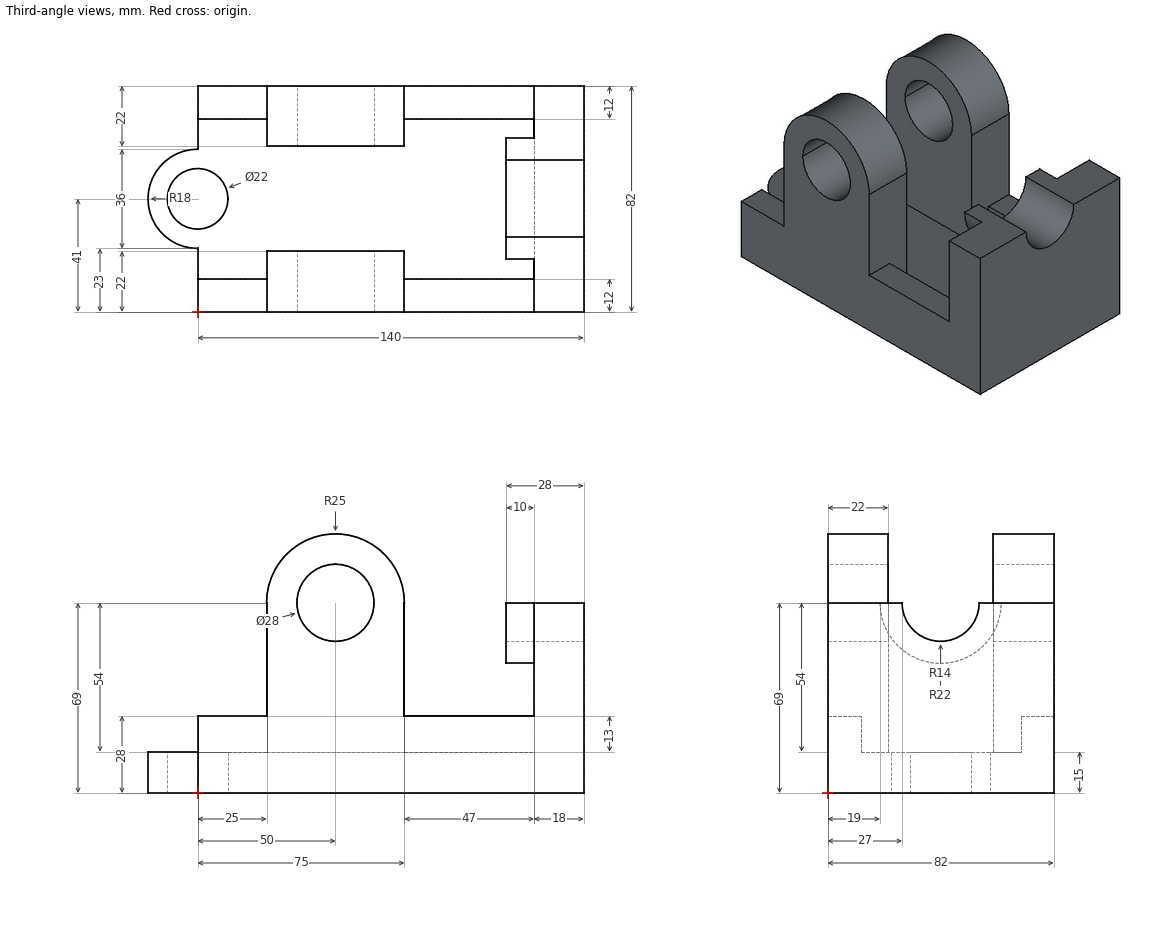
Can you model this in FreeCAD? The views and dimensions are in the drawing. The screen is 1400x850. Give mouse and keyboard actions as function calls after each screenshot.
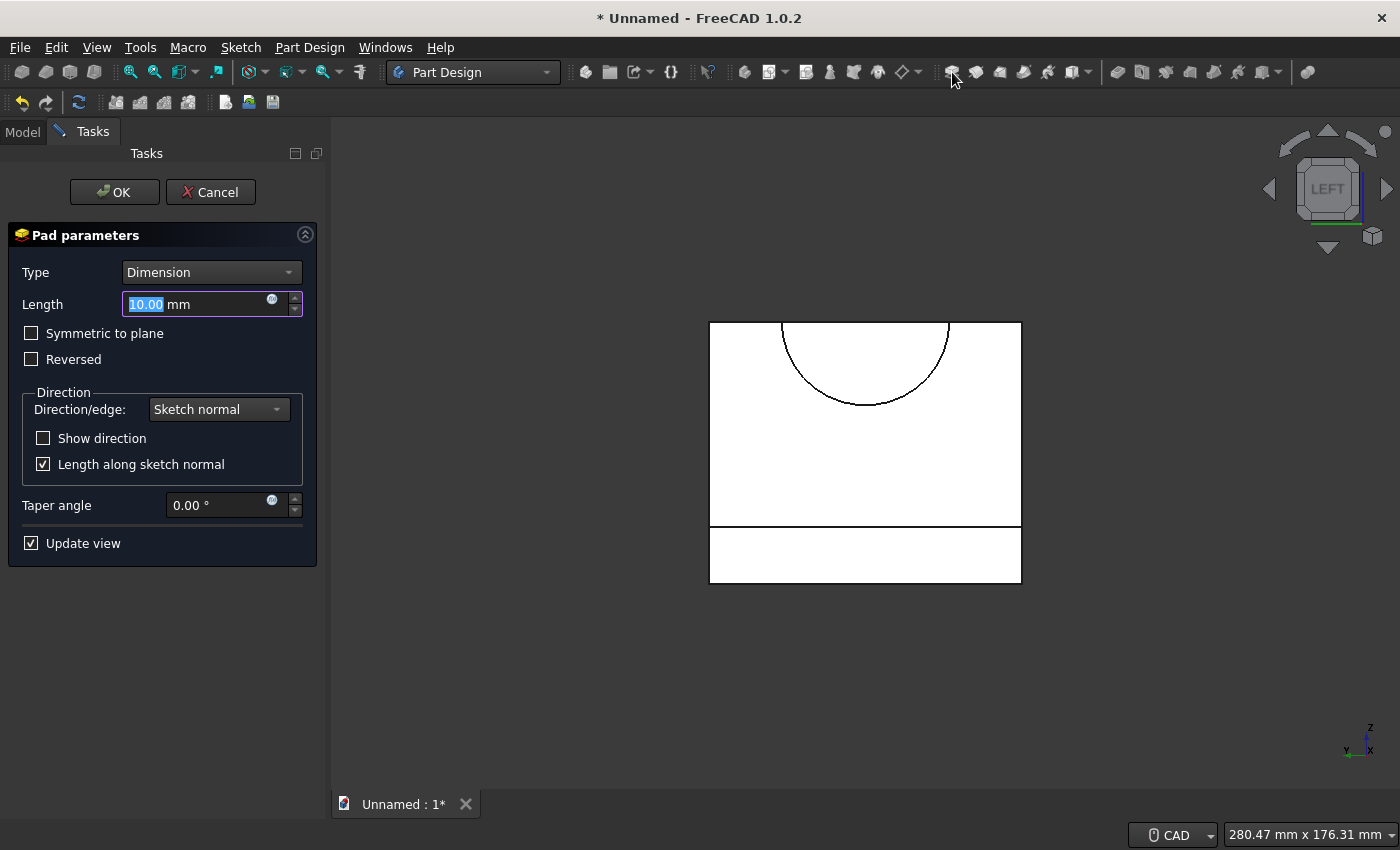
text(10)
key(Tab)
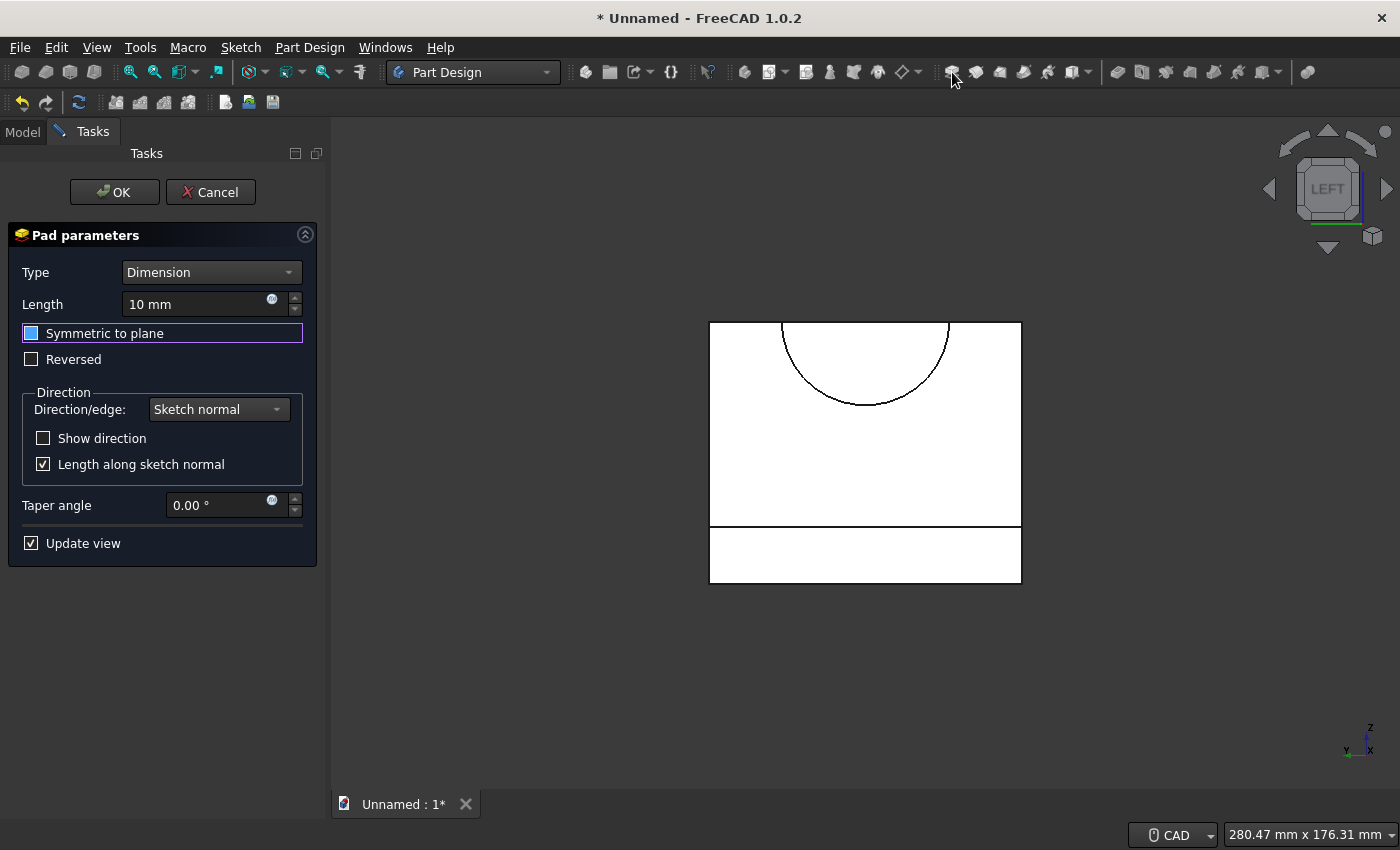
click(115, 192)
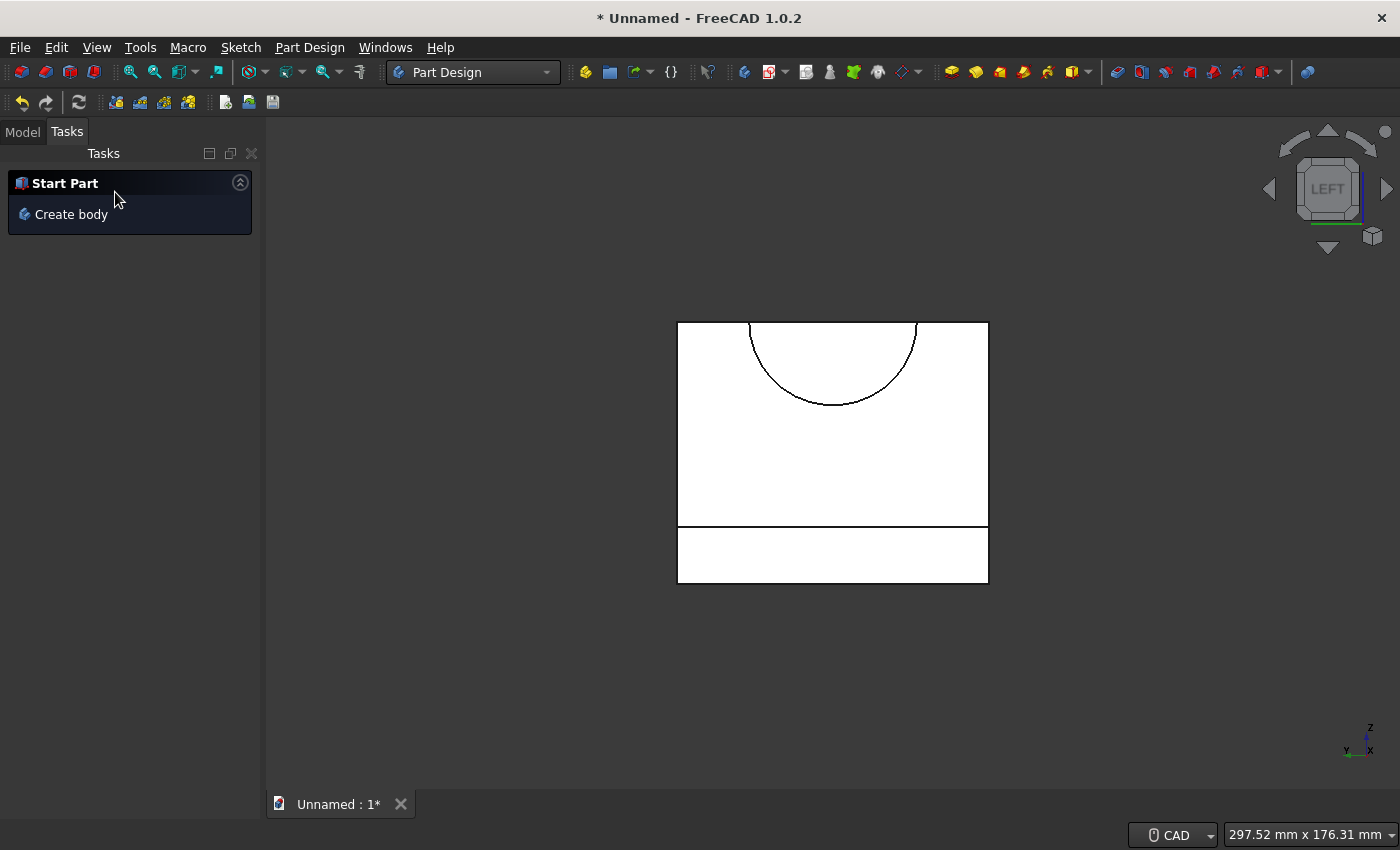
click(132, 72)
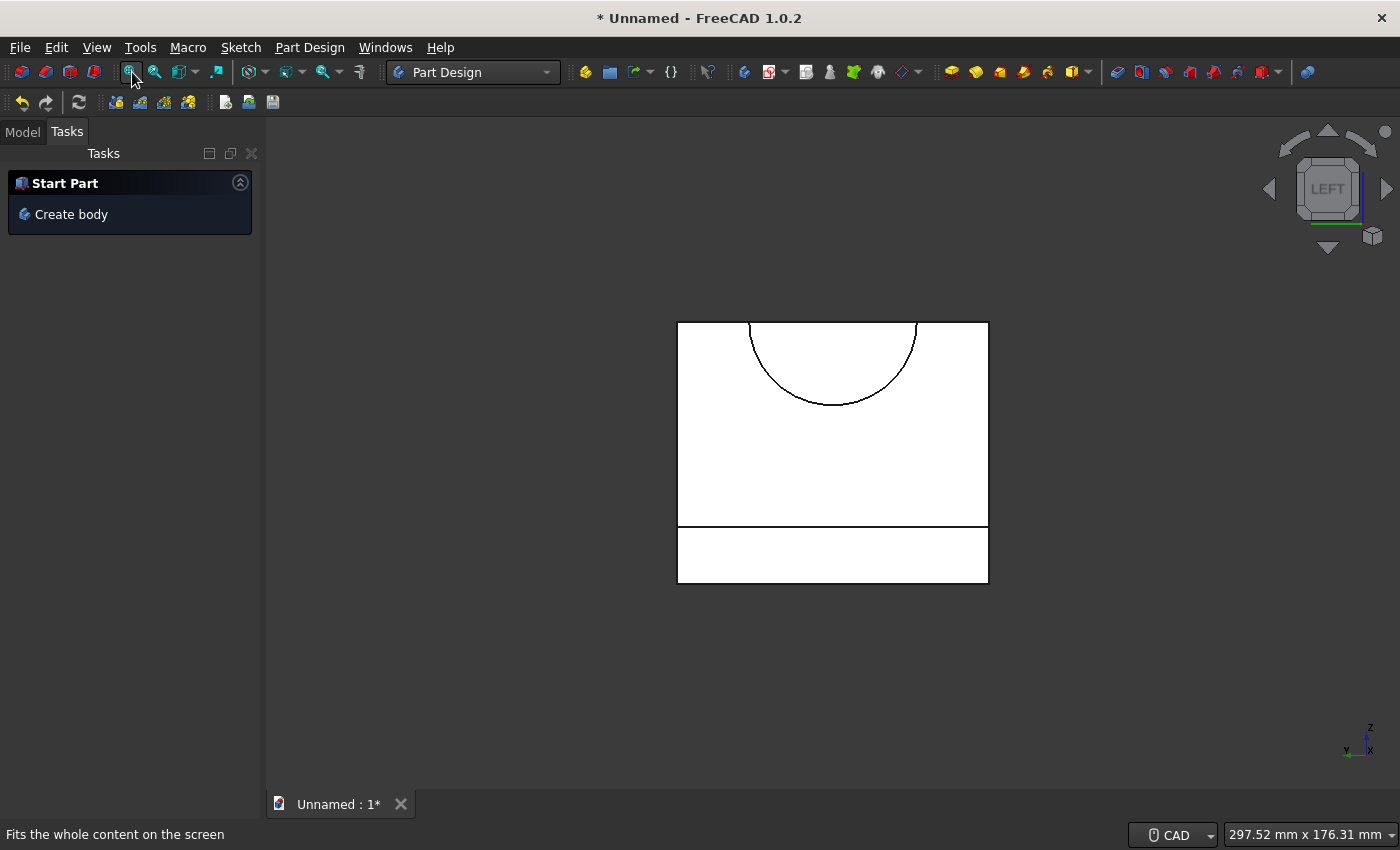
click(833, 362)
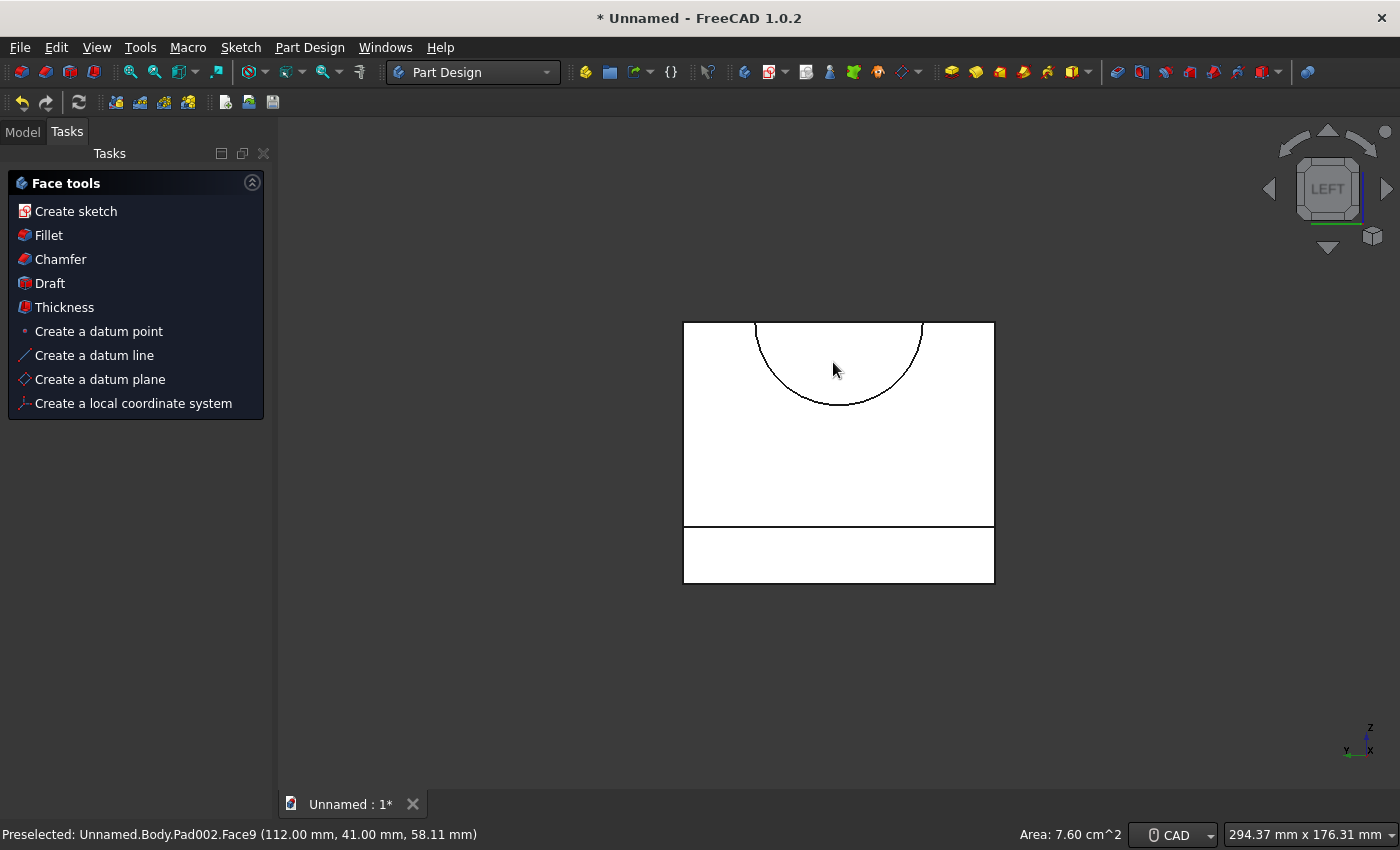
click(770, 72)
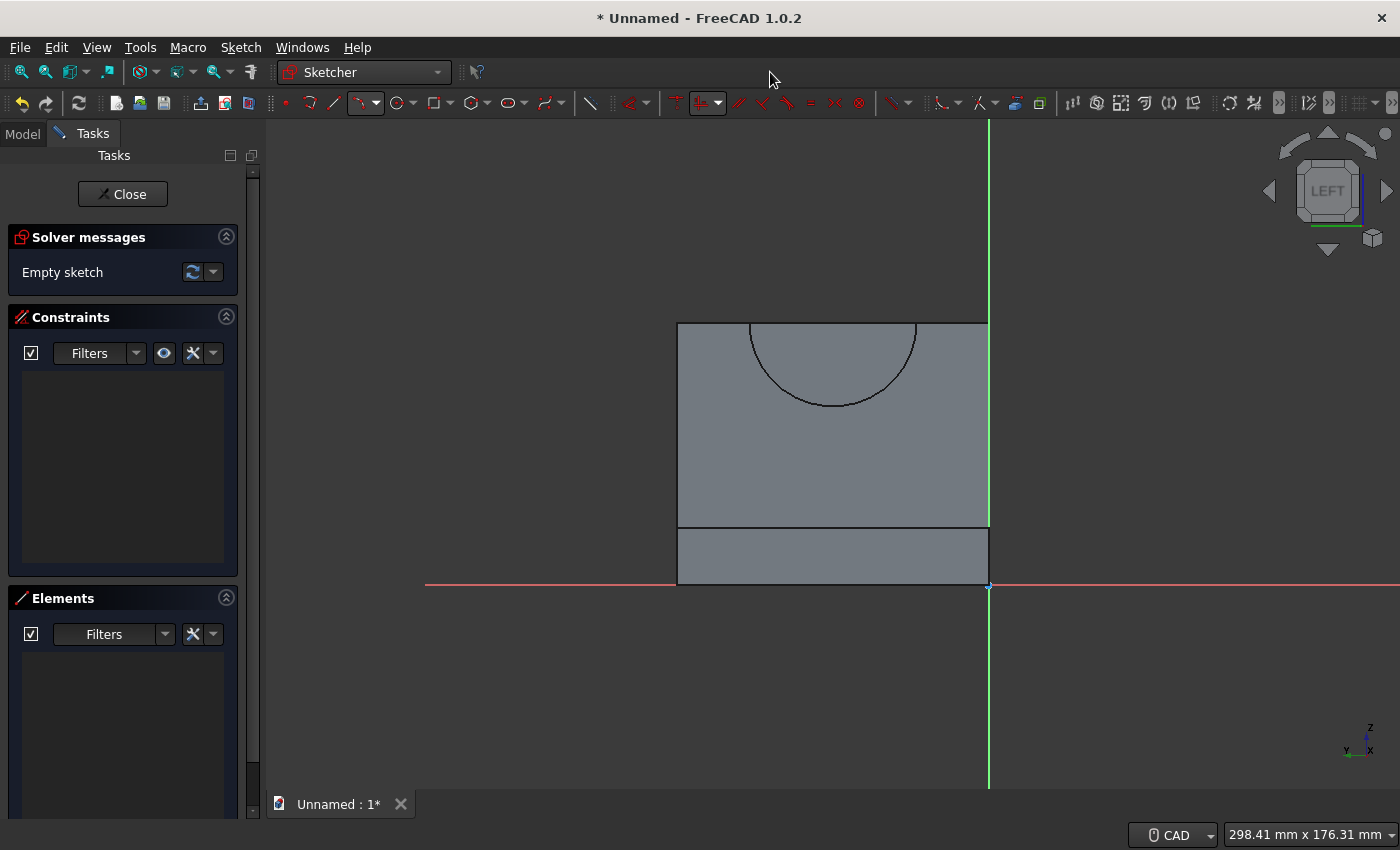
click(250, 104)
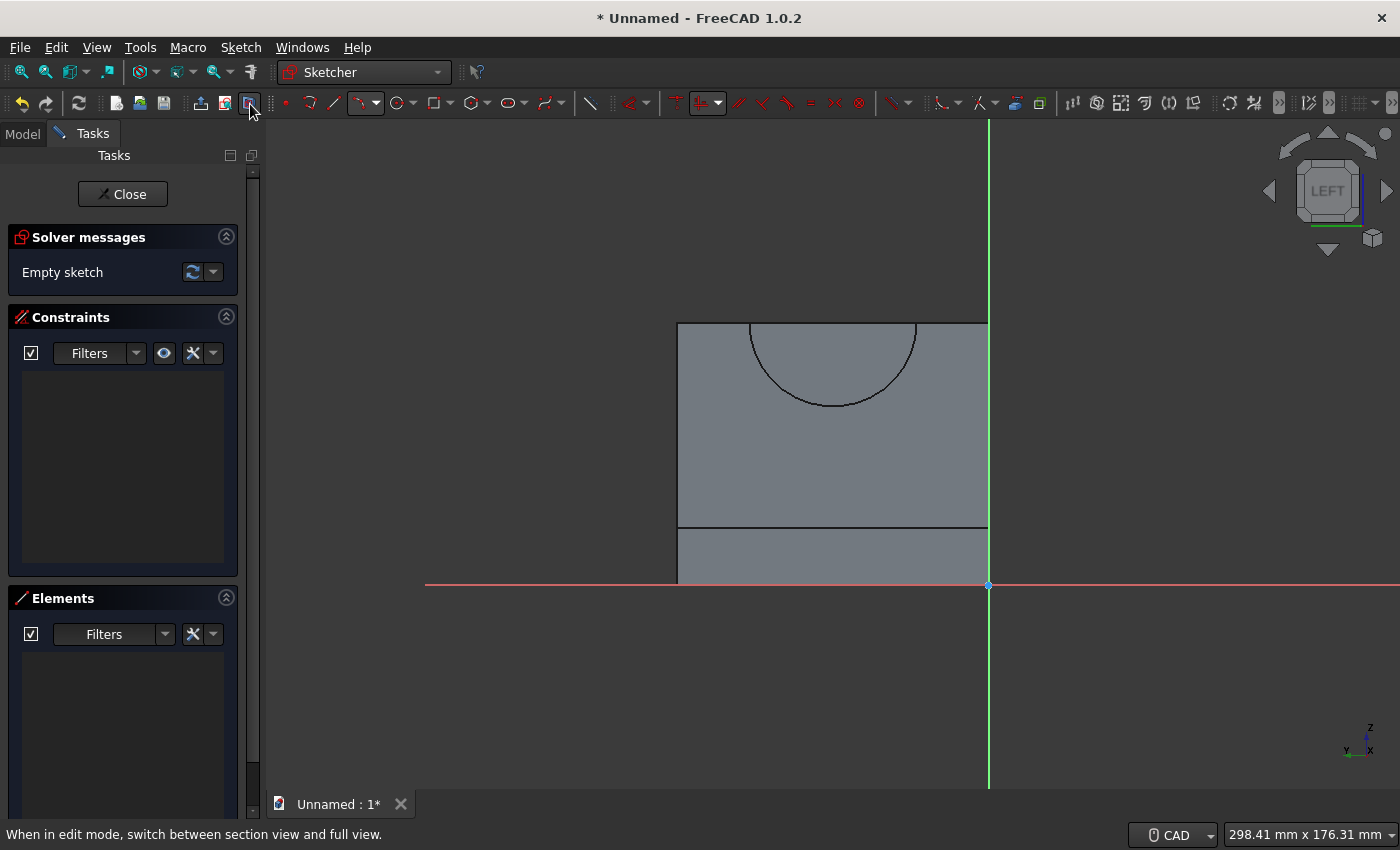
scroll(1030, 454, up, 3)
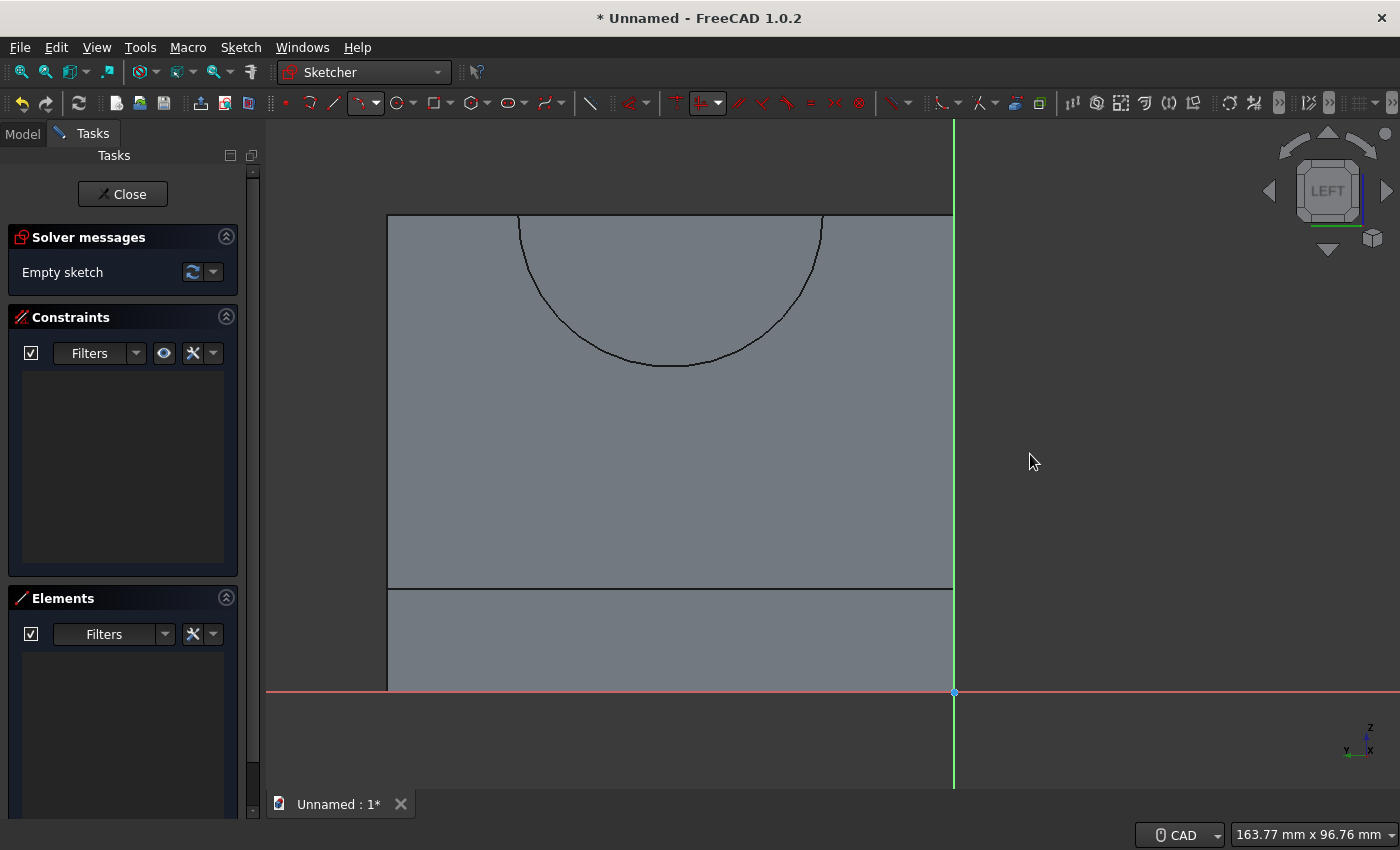
click(334, 104)